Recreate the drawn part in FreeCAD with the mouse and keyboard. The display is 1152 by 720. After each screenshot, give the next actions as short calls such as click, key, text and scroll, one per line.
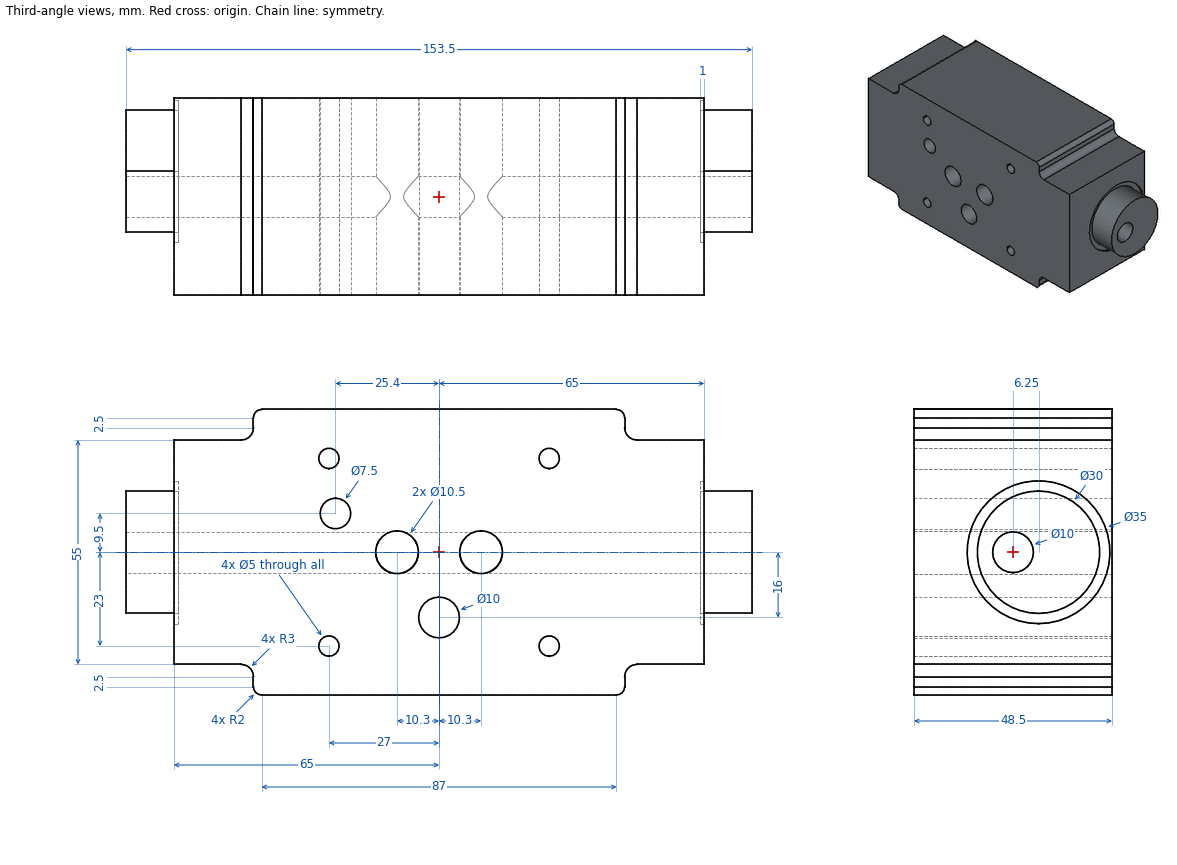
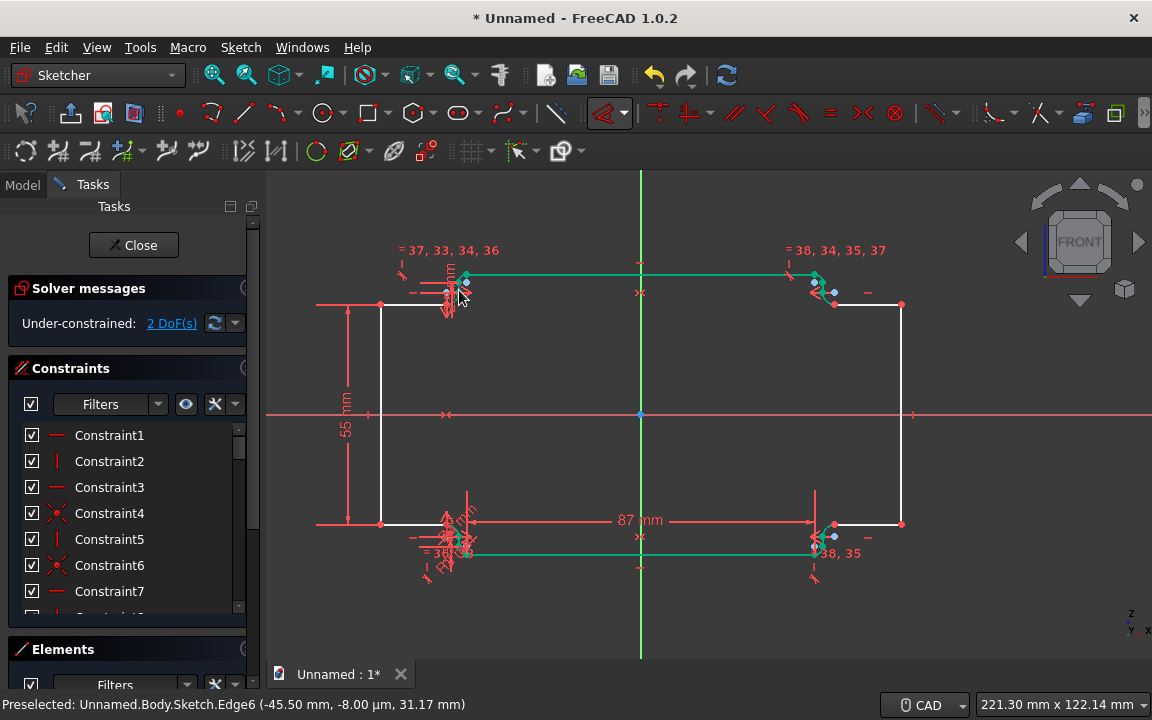
click(381, 525)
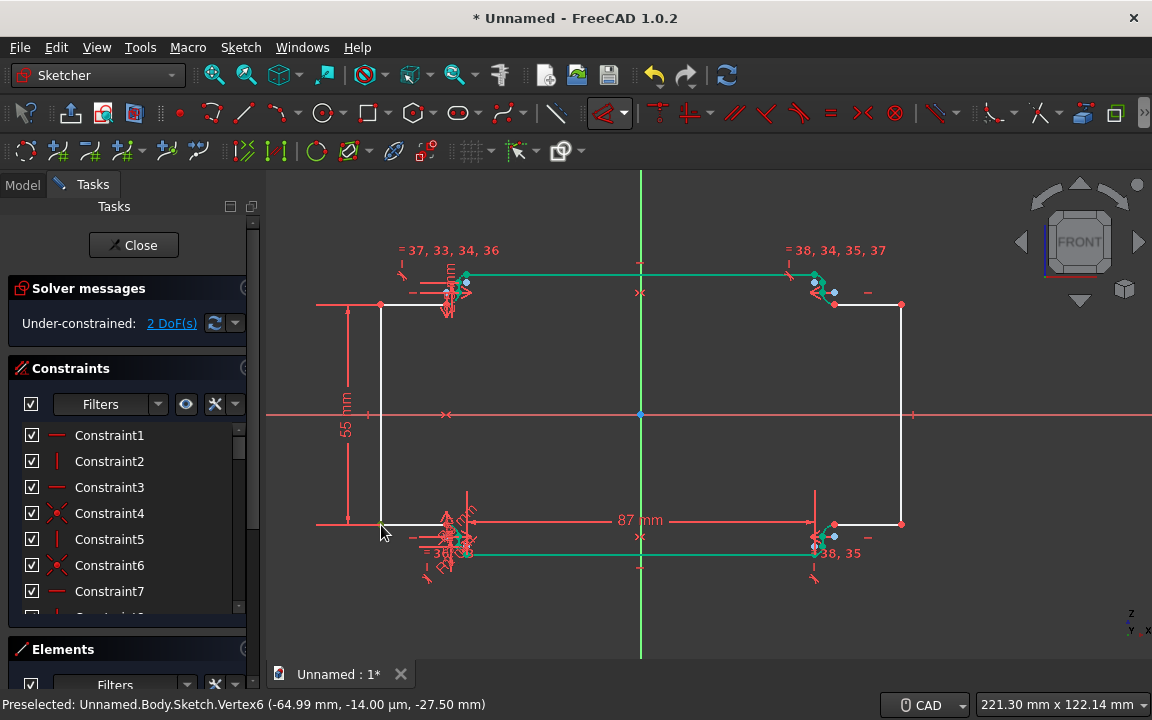
click(626, 114)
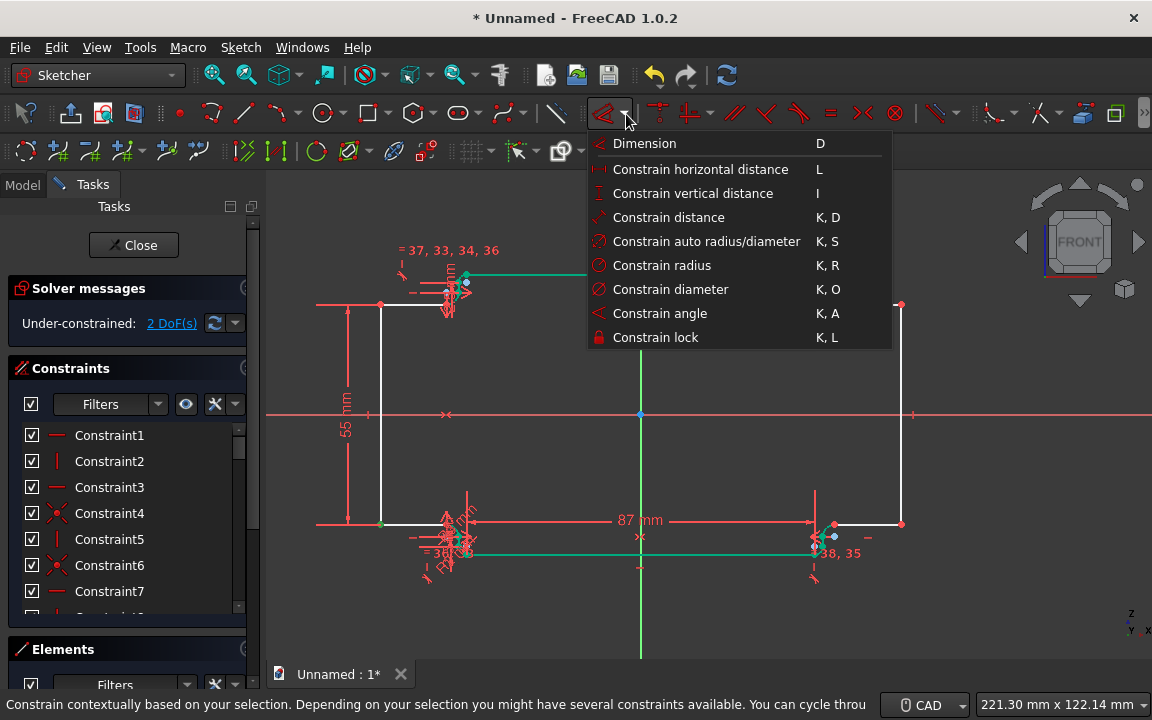
click(740, 169)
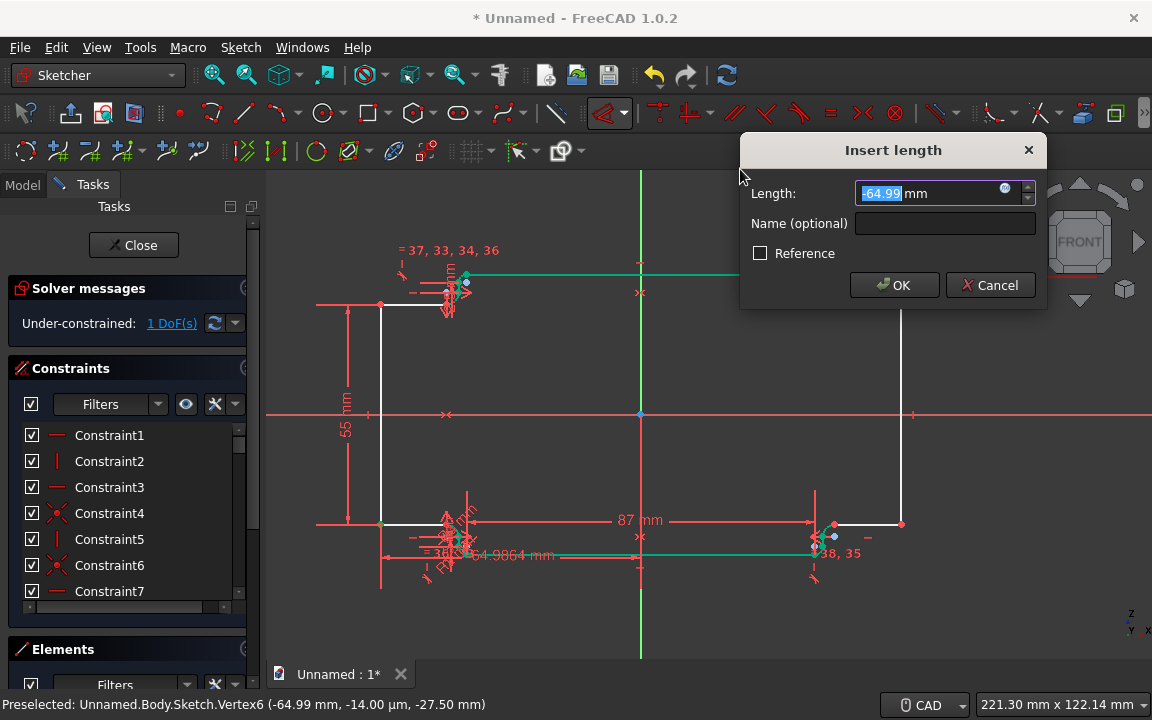
text(-65)
key(Return)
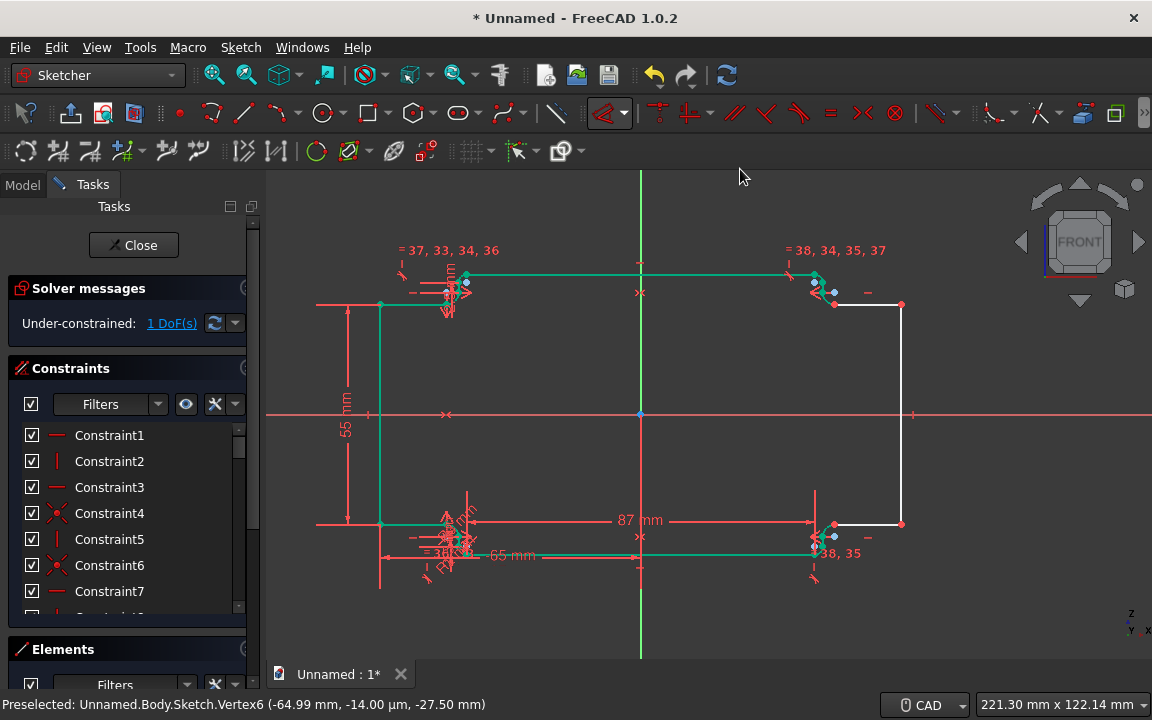
click(901, 305)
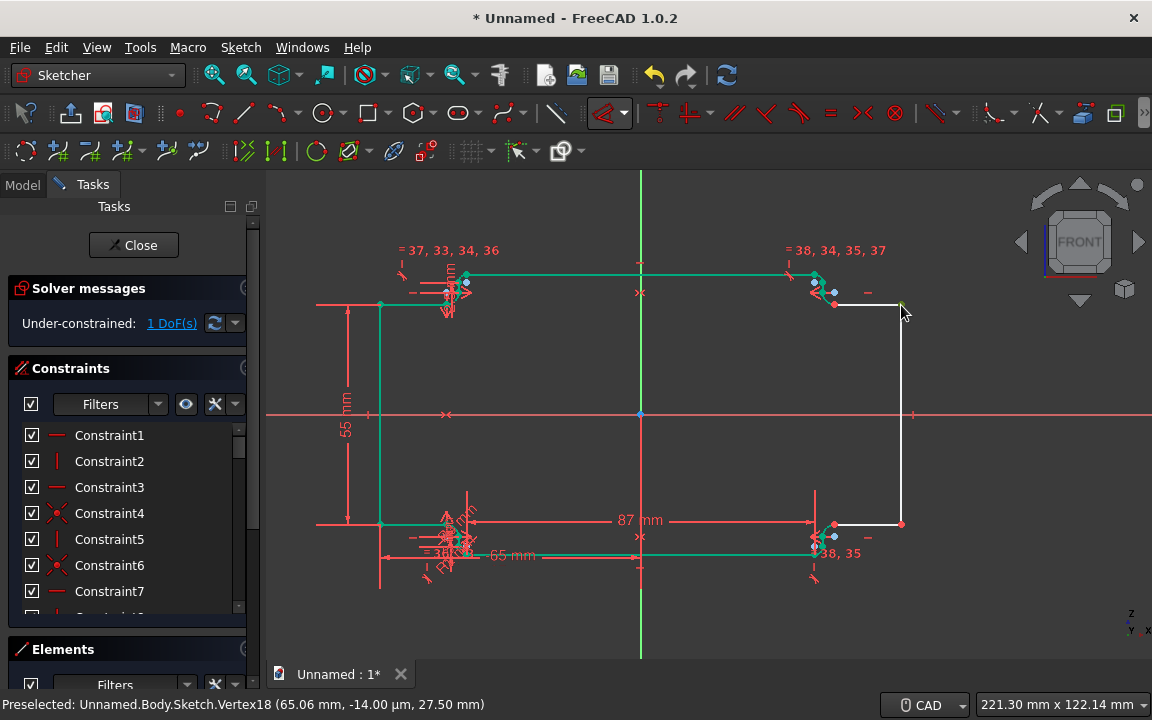
key(l)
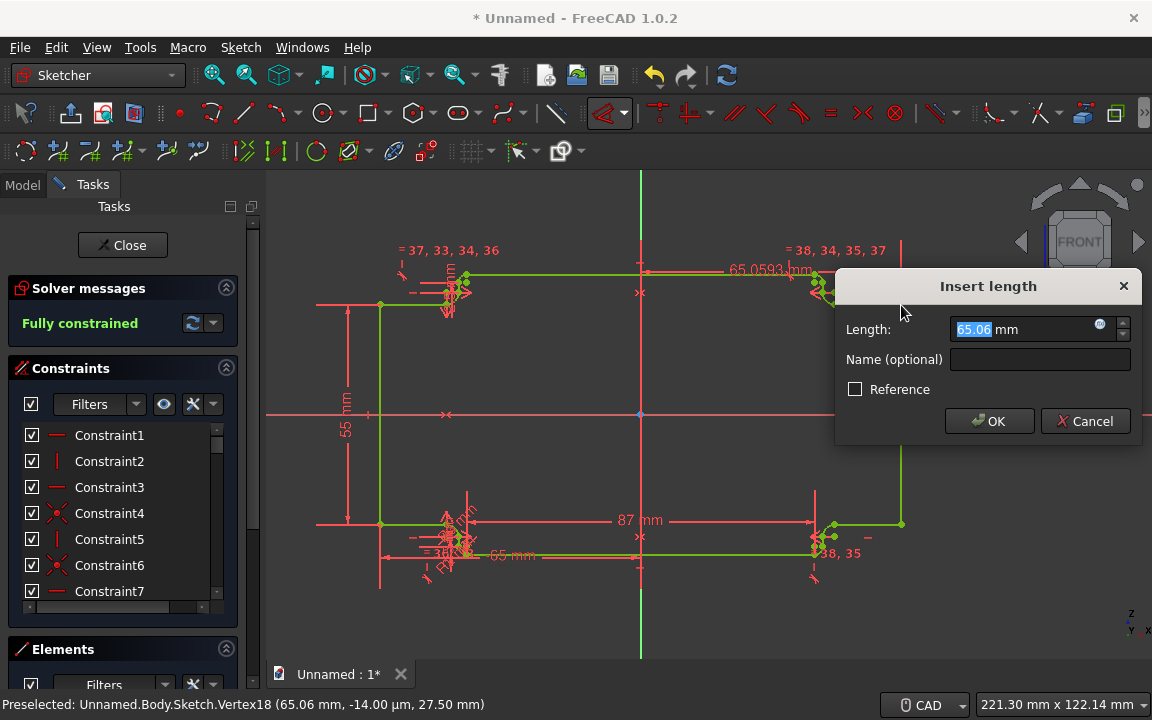
text(65)
key(Return)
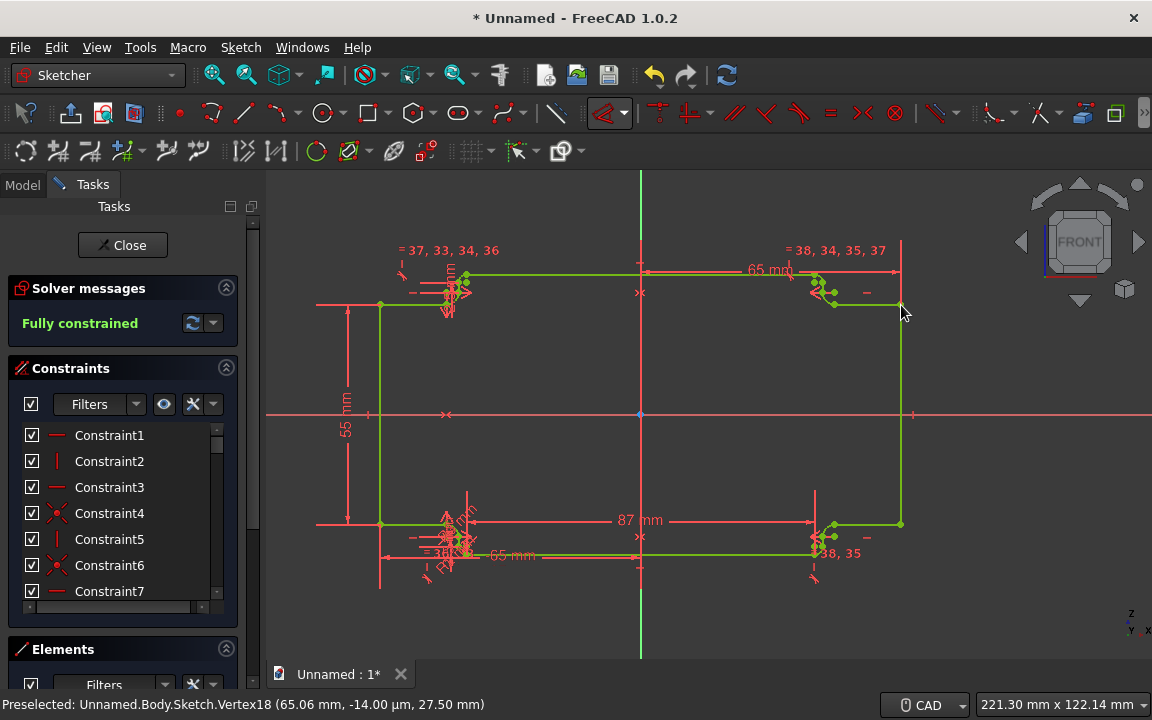
click(123, 245)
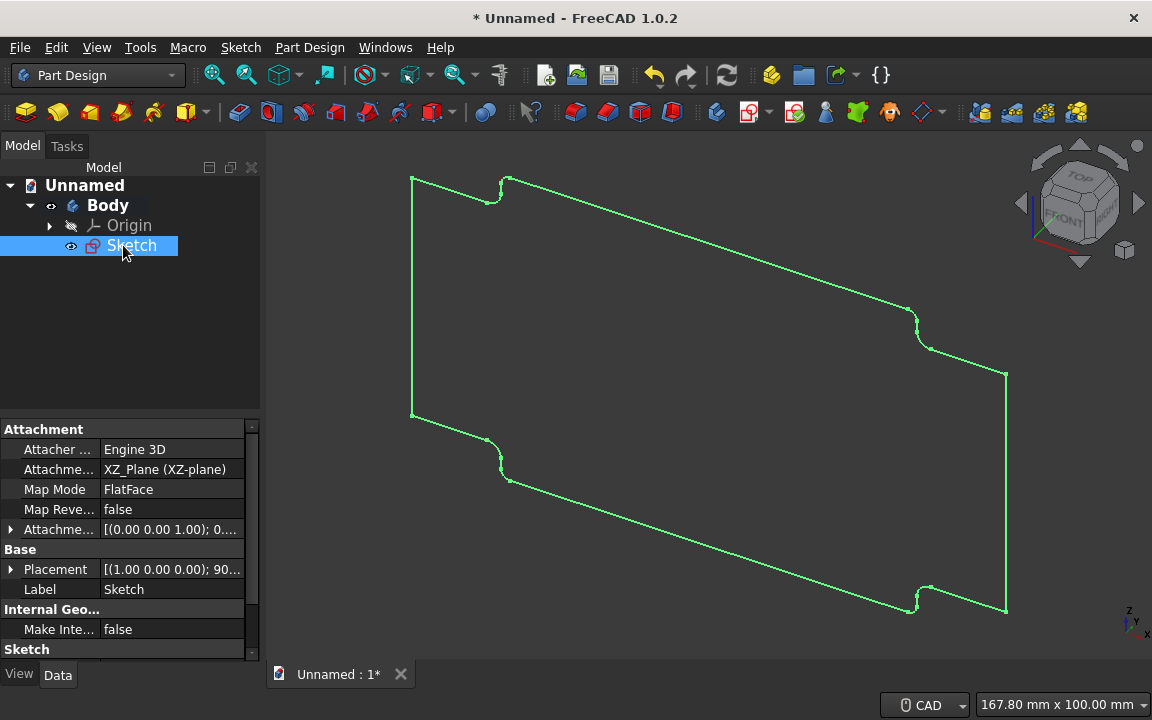
click(26, 112)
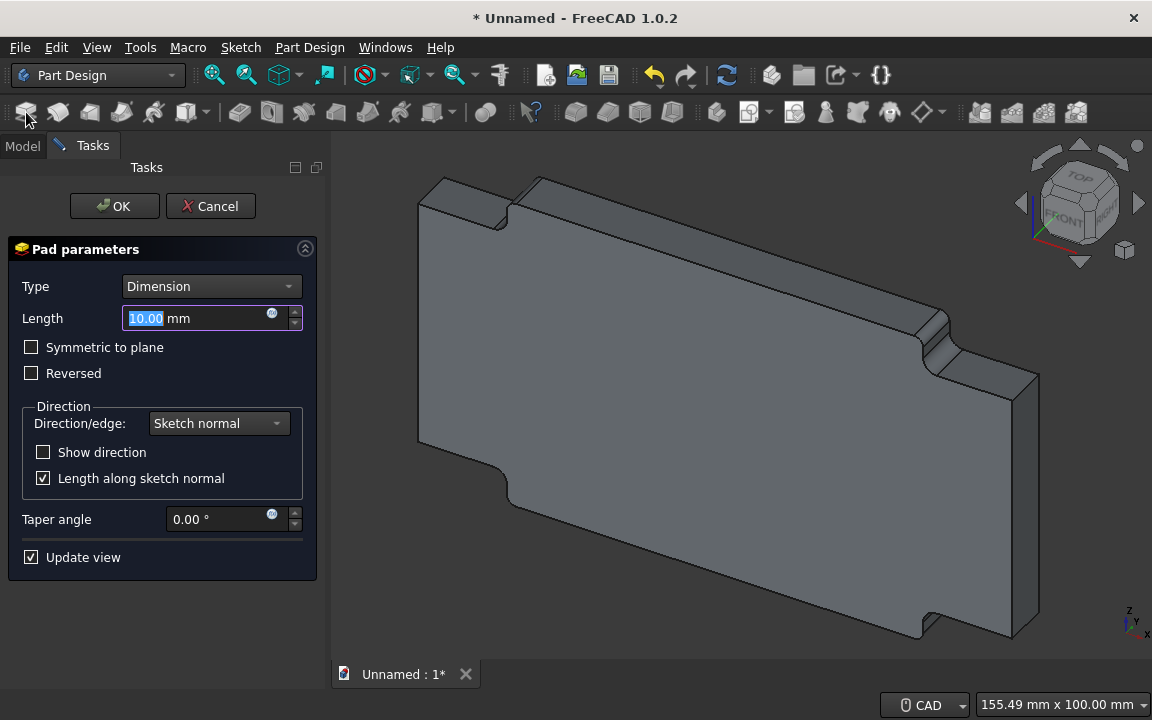
text(48.5)
key(Tab)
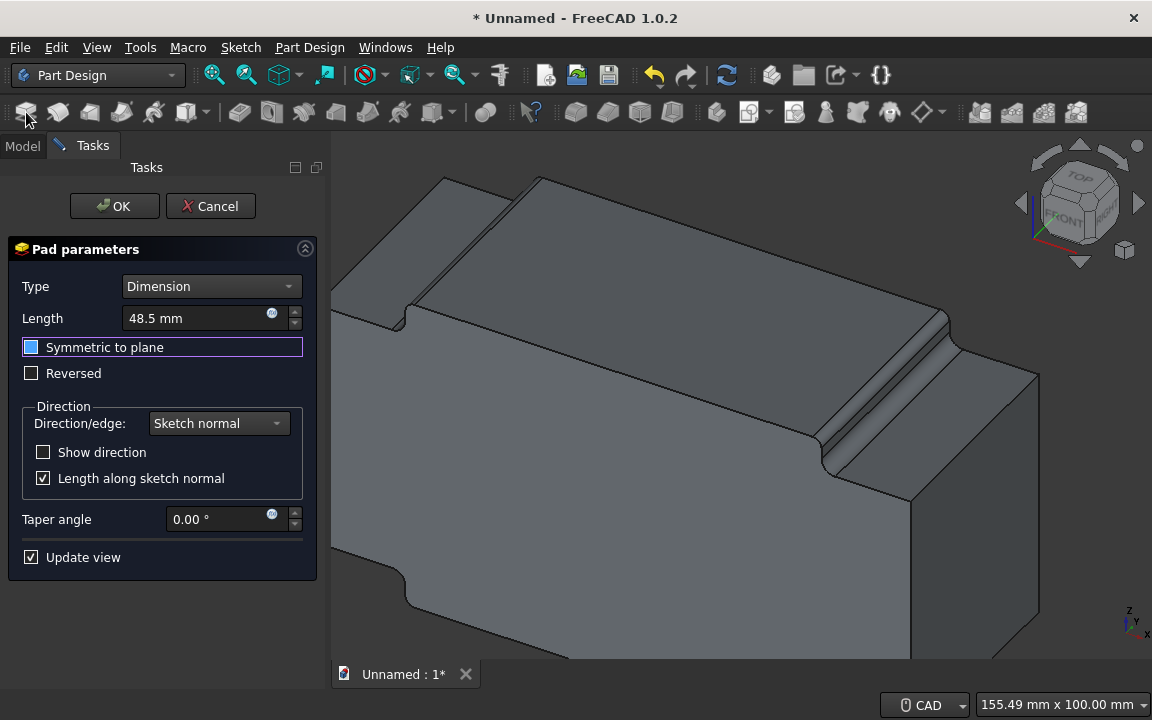
click(30, 347)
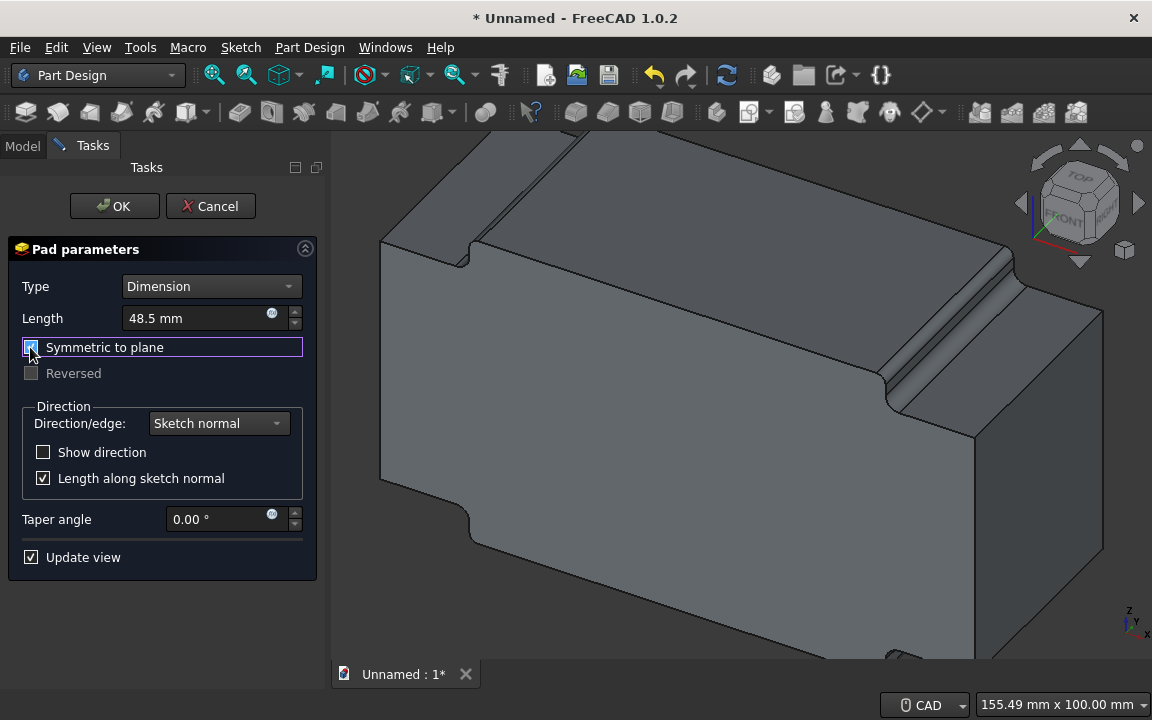
click(115, 206)